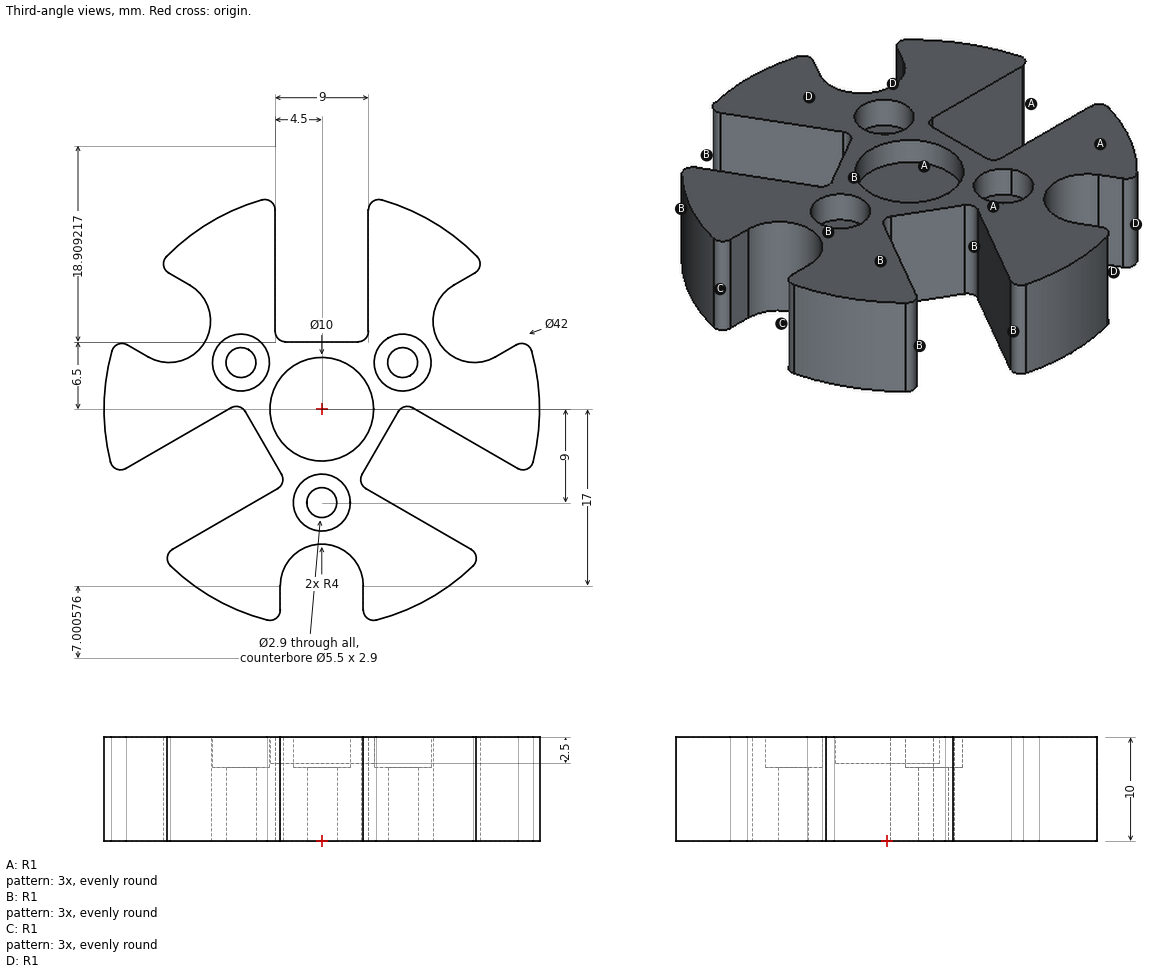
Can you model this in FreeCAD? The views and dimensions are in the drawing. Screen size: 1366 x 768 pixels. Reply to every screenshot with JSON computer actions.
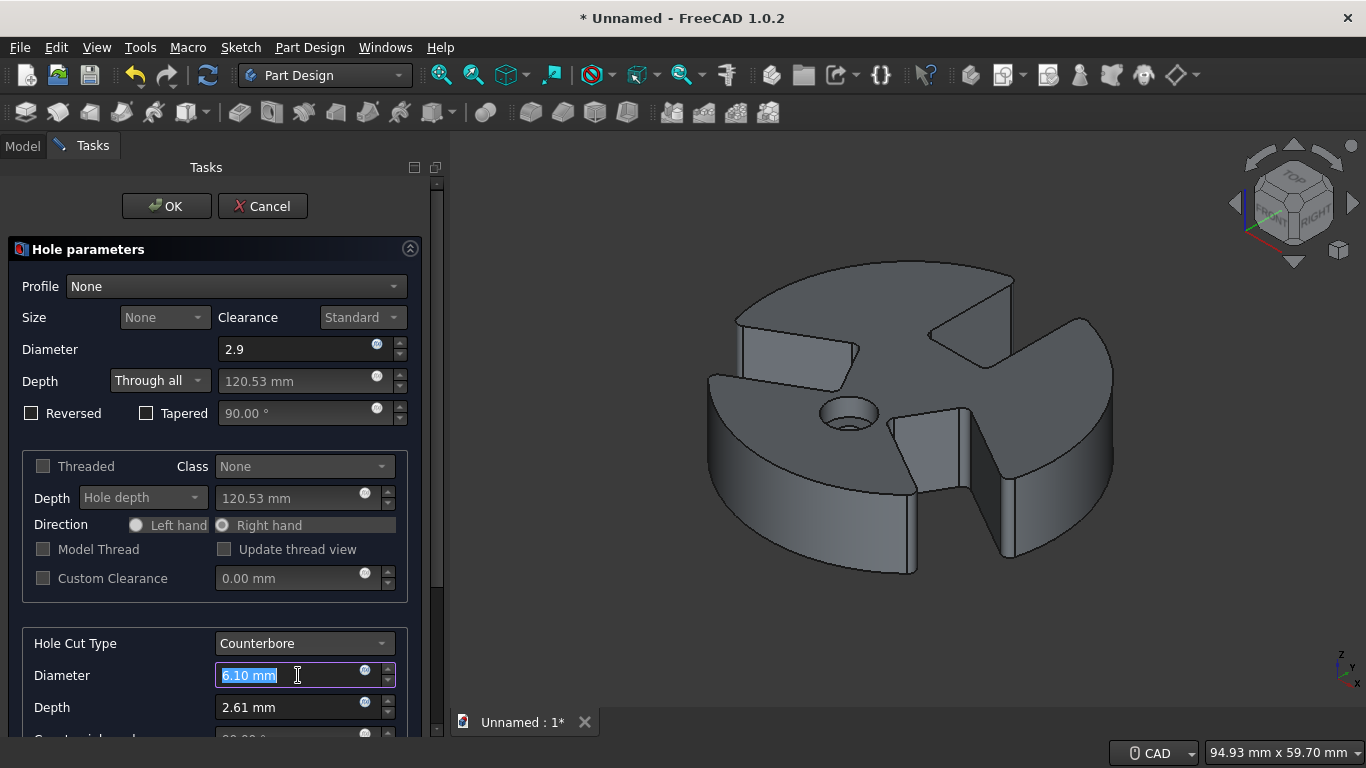
{"action": "type", "text": "5.5"}
{"action": "key", "text": "Tab"}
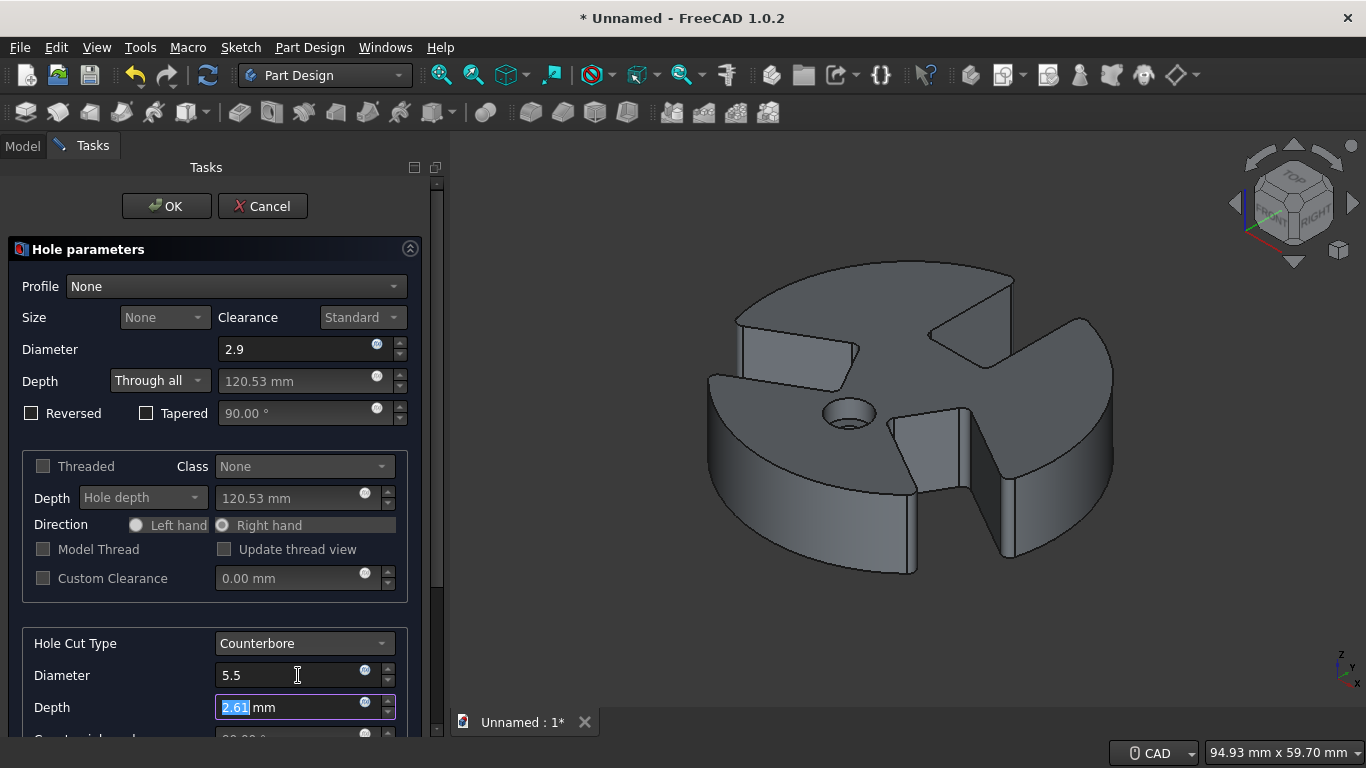
{"action": "type", "text": "2.9"}
{"action": "key", "text": "Tab"}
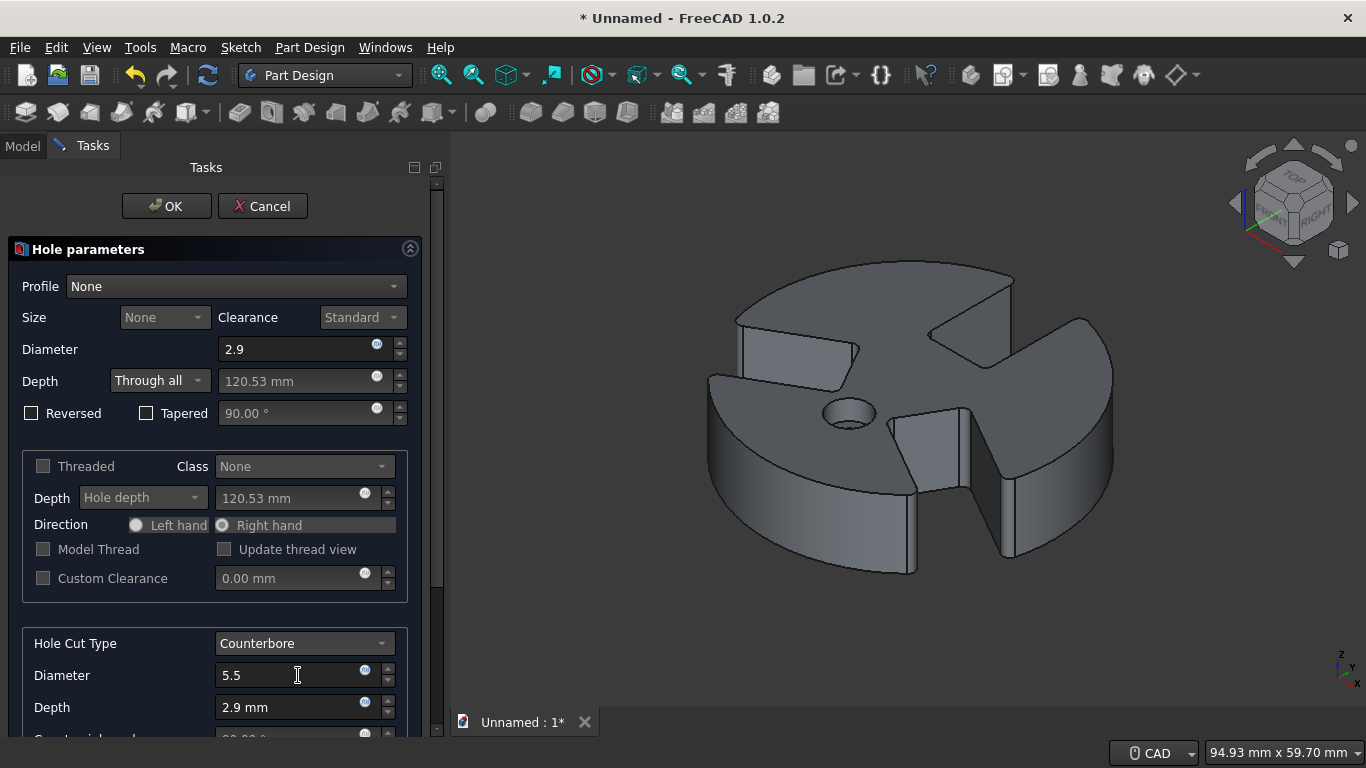
{"action": "left_click", "coordinate": [167, 206]}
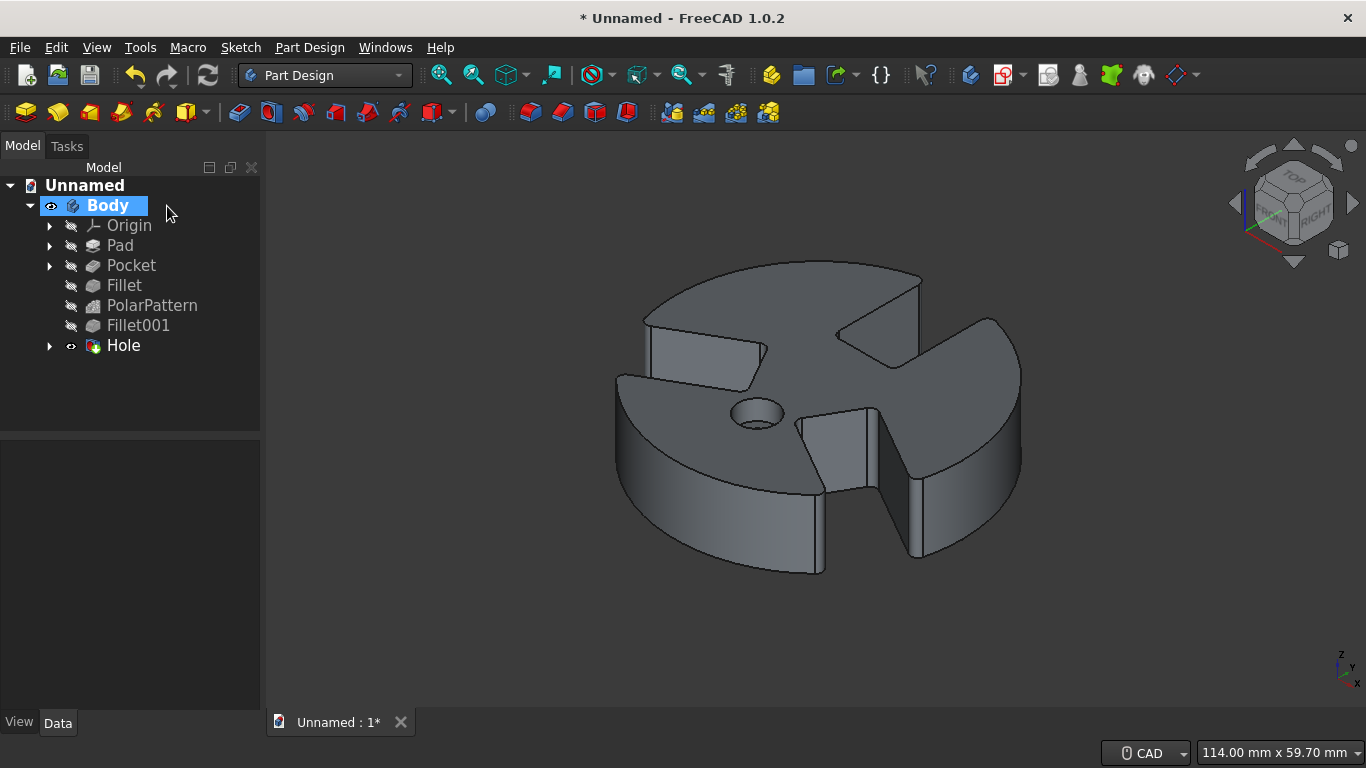
{"action": "left_click", "coordinate": [116, 346]}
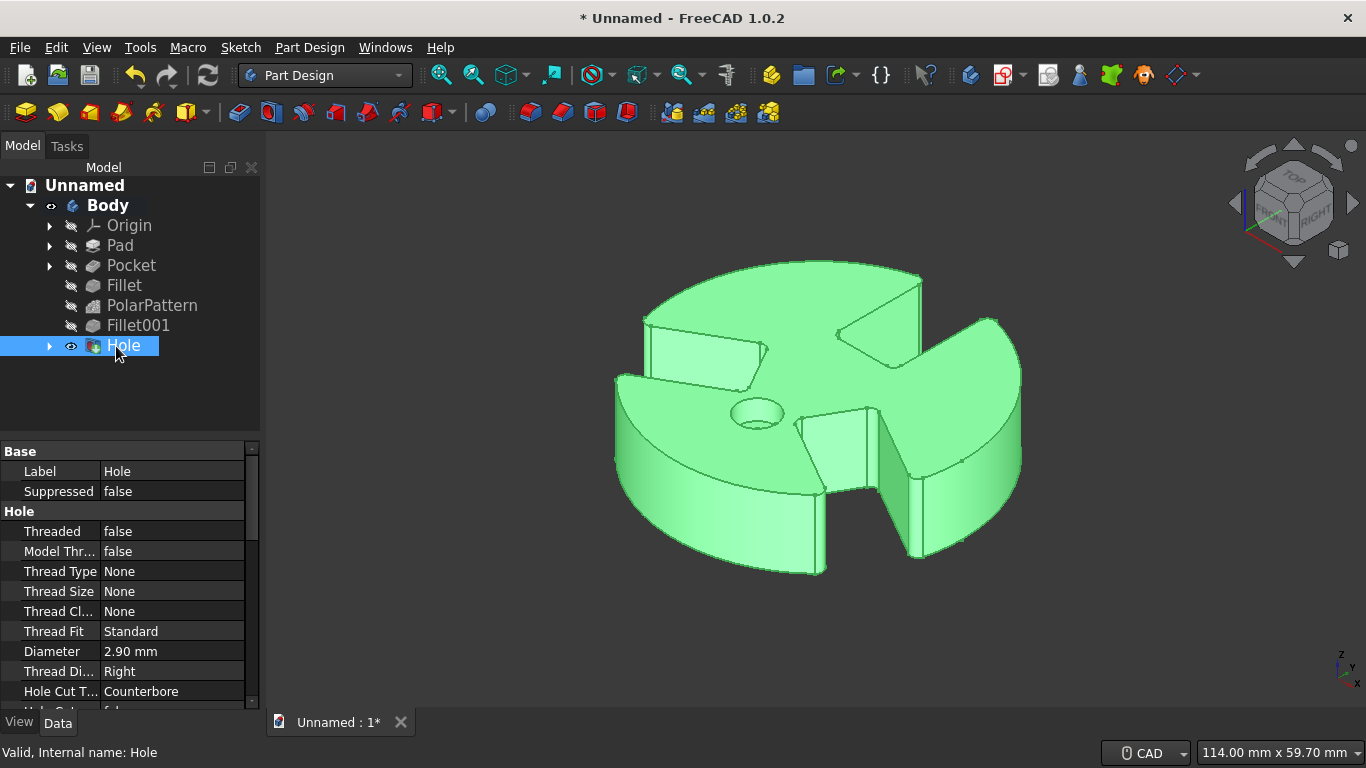
{"action": "left_click", "coordinate": [736, 112]}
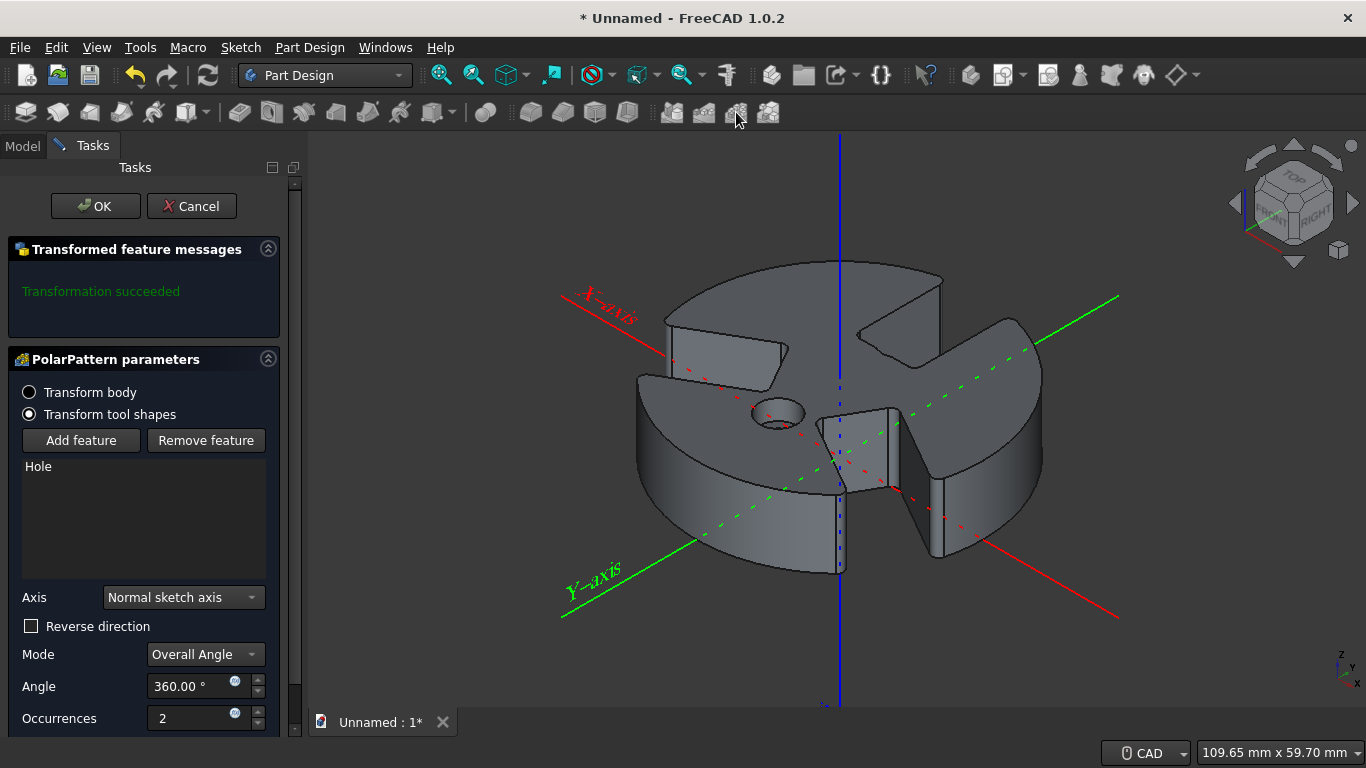
{"action": "left_click", "coordinate": [184, 598]}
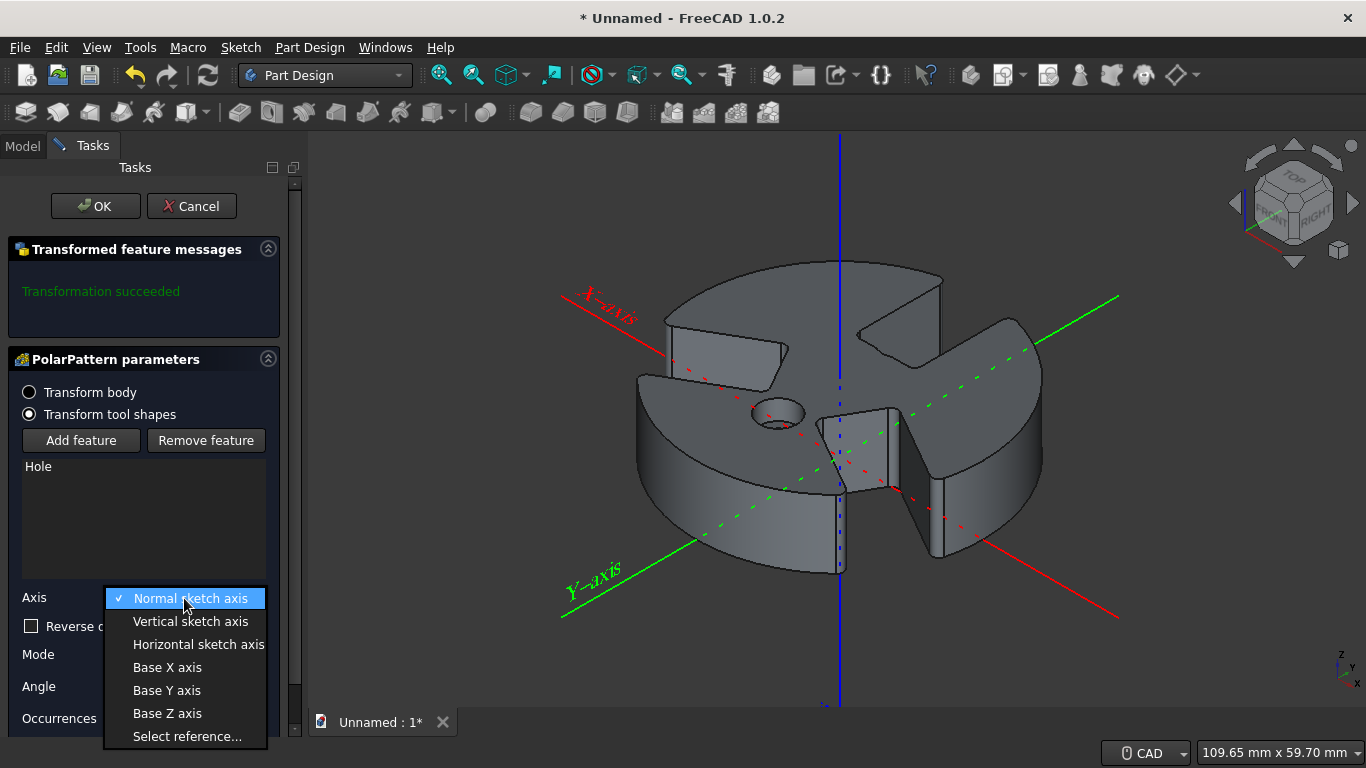
{"action": "left_click", "coordinate": [184, 714]}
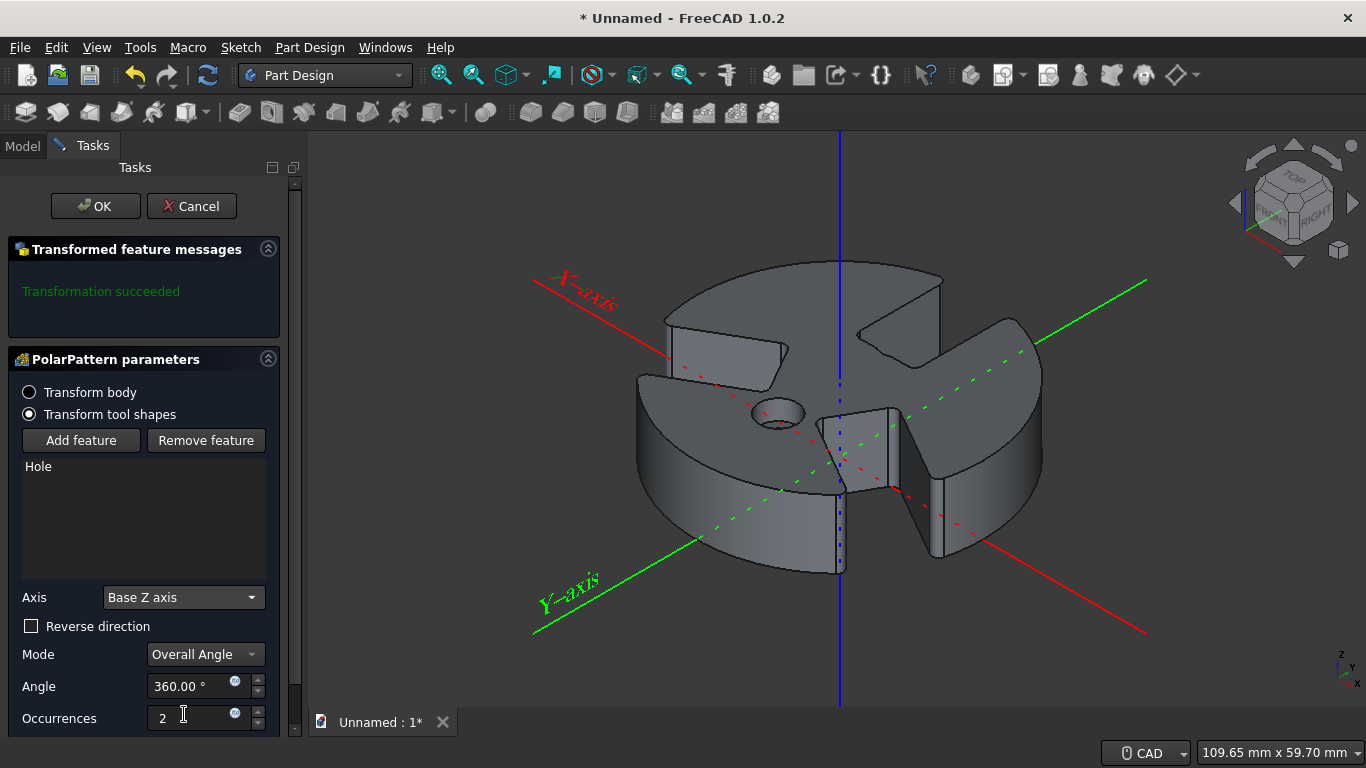
{"action": "triple_click", "coordinate": [198, 718]}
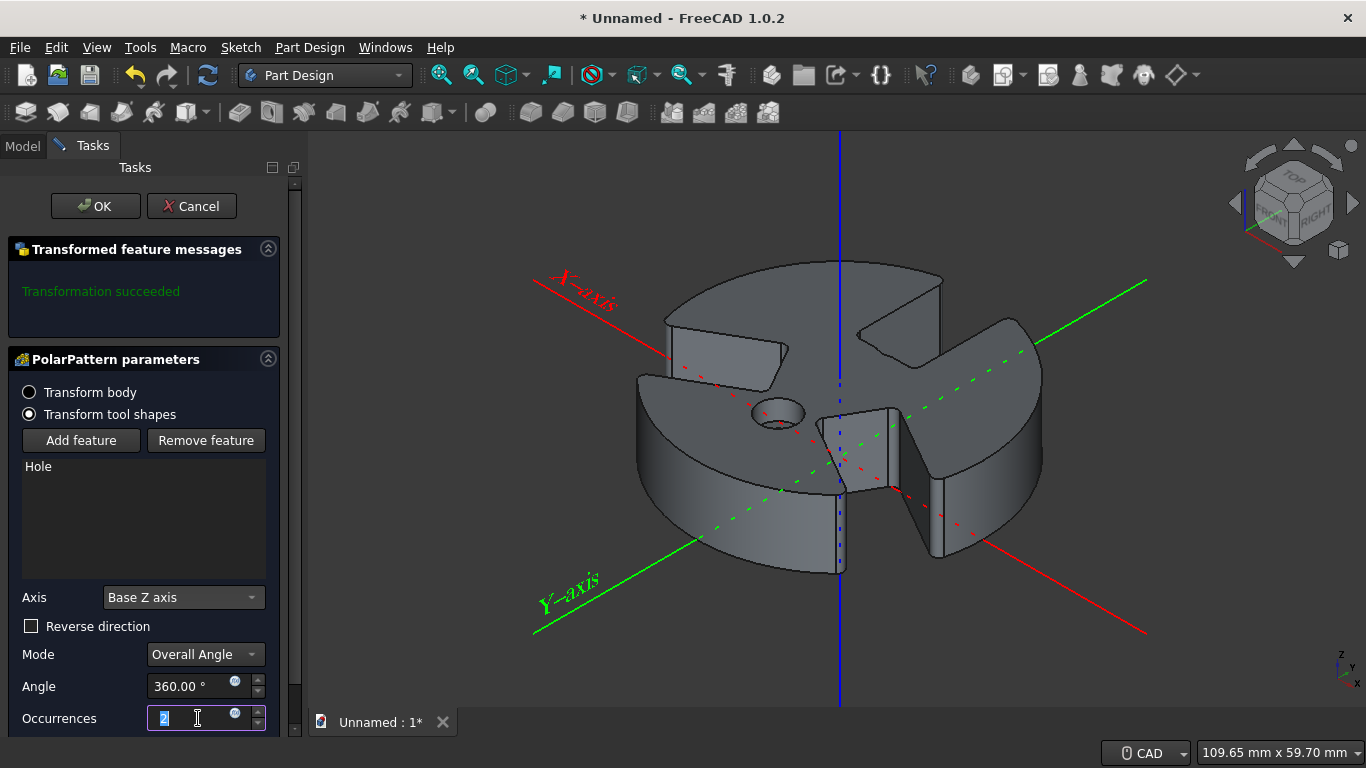
{"action": "type", "text": "3"}
{"action": "key", "text": "Tab"}